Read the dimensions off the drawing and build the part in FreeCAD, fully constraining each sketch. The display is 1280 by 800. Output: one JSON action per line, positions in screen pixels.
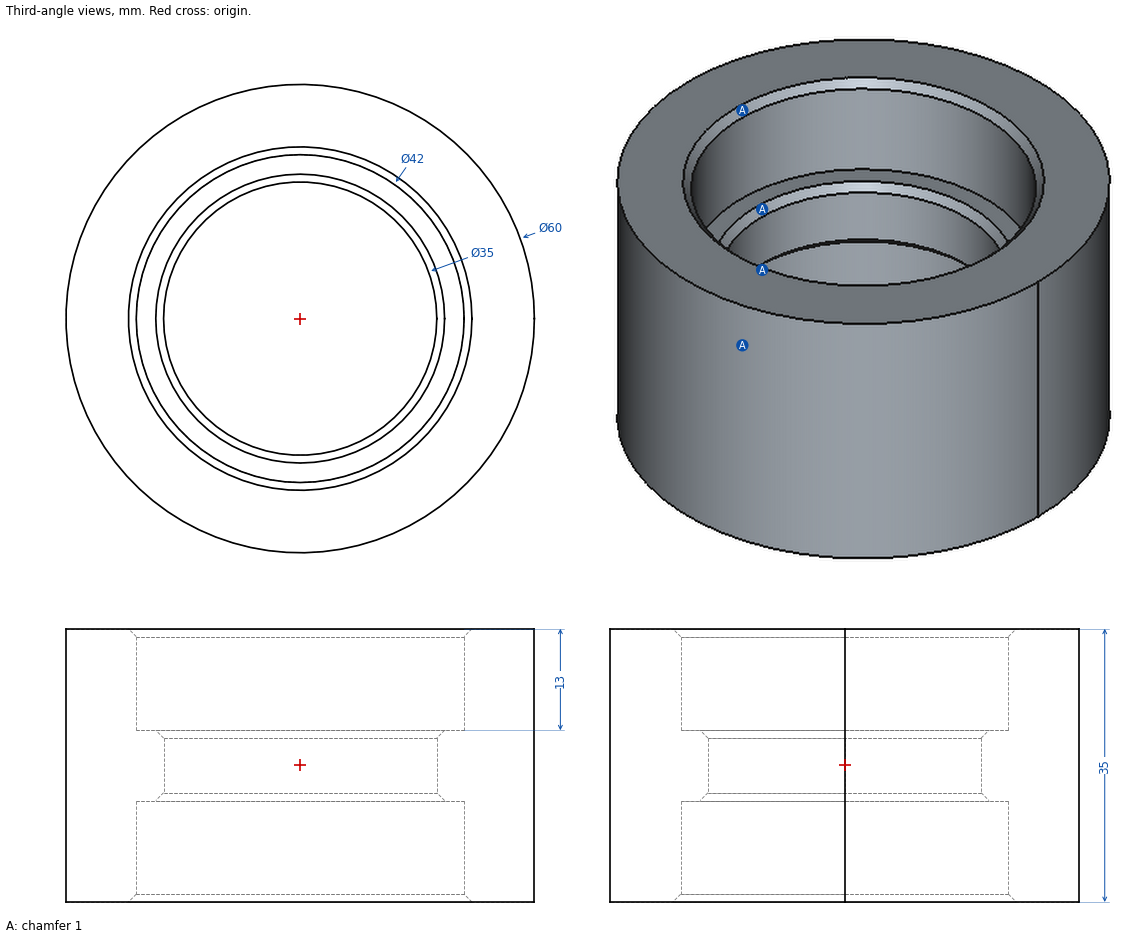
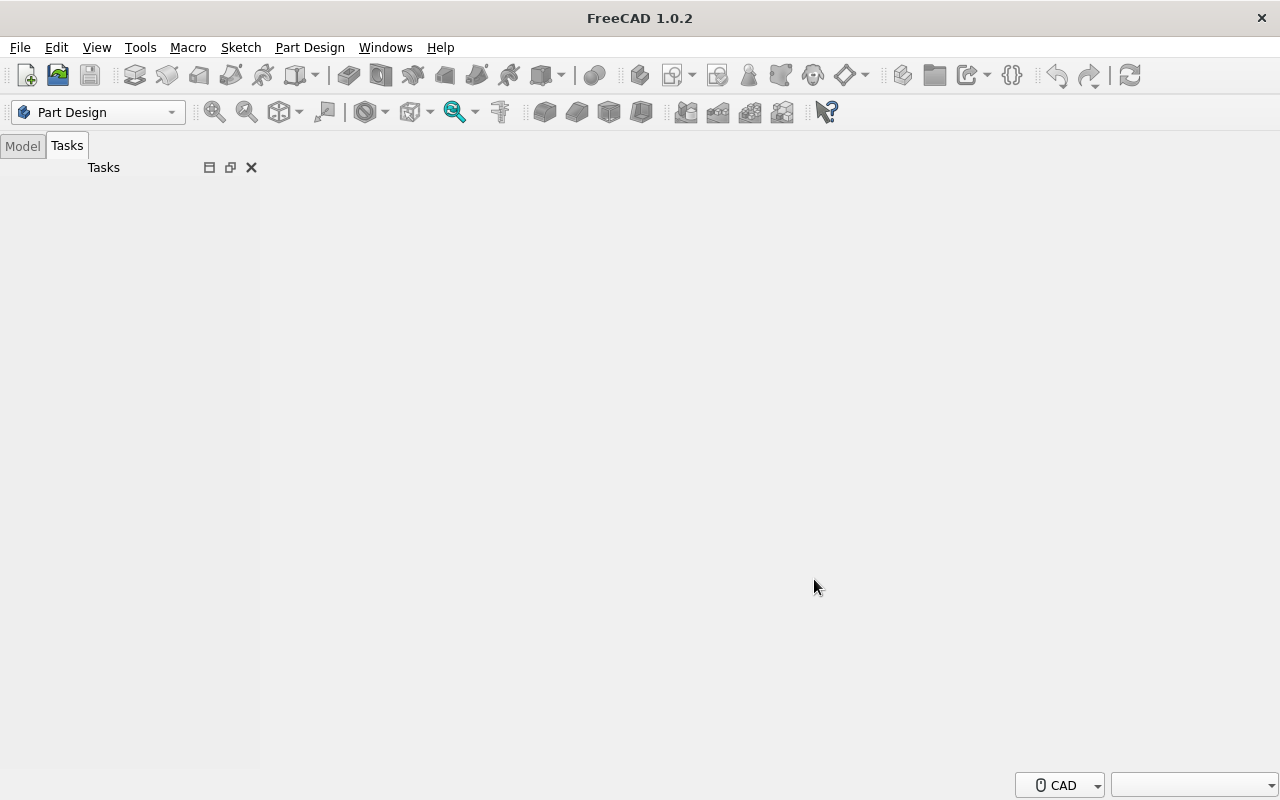
{"action": "left_click", "coordinate": [26, 76]}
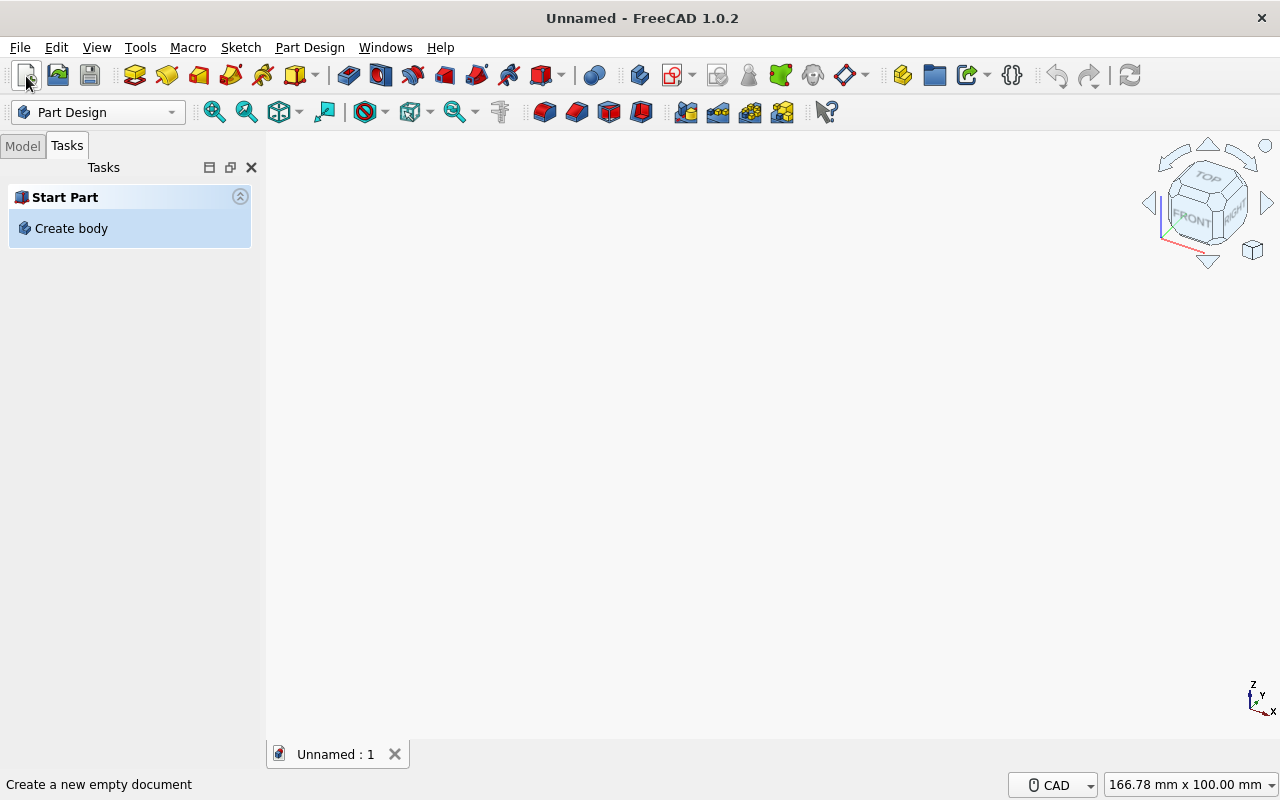
{"action": "left_click", "coordinate": [672, 76]}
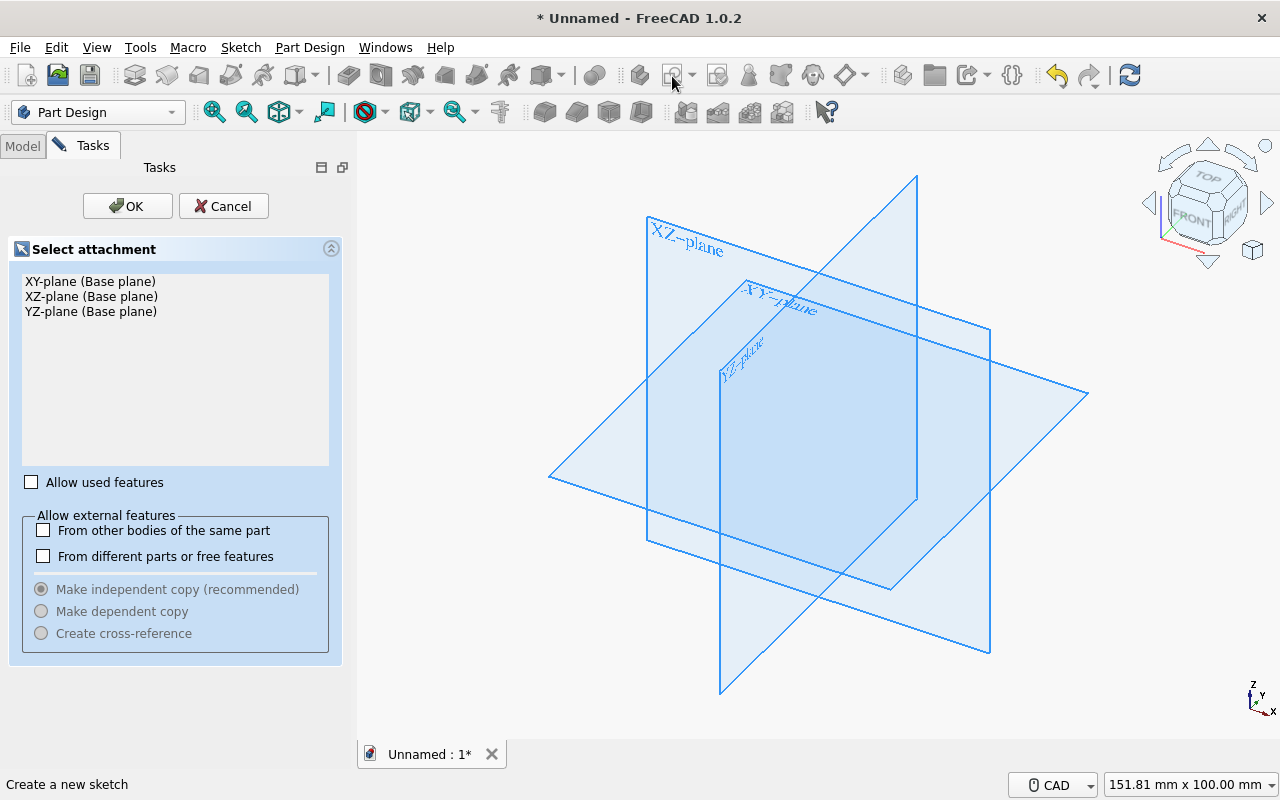
{"action": "left_click", "coordinate": [82, 282]}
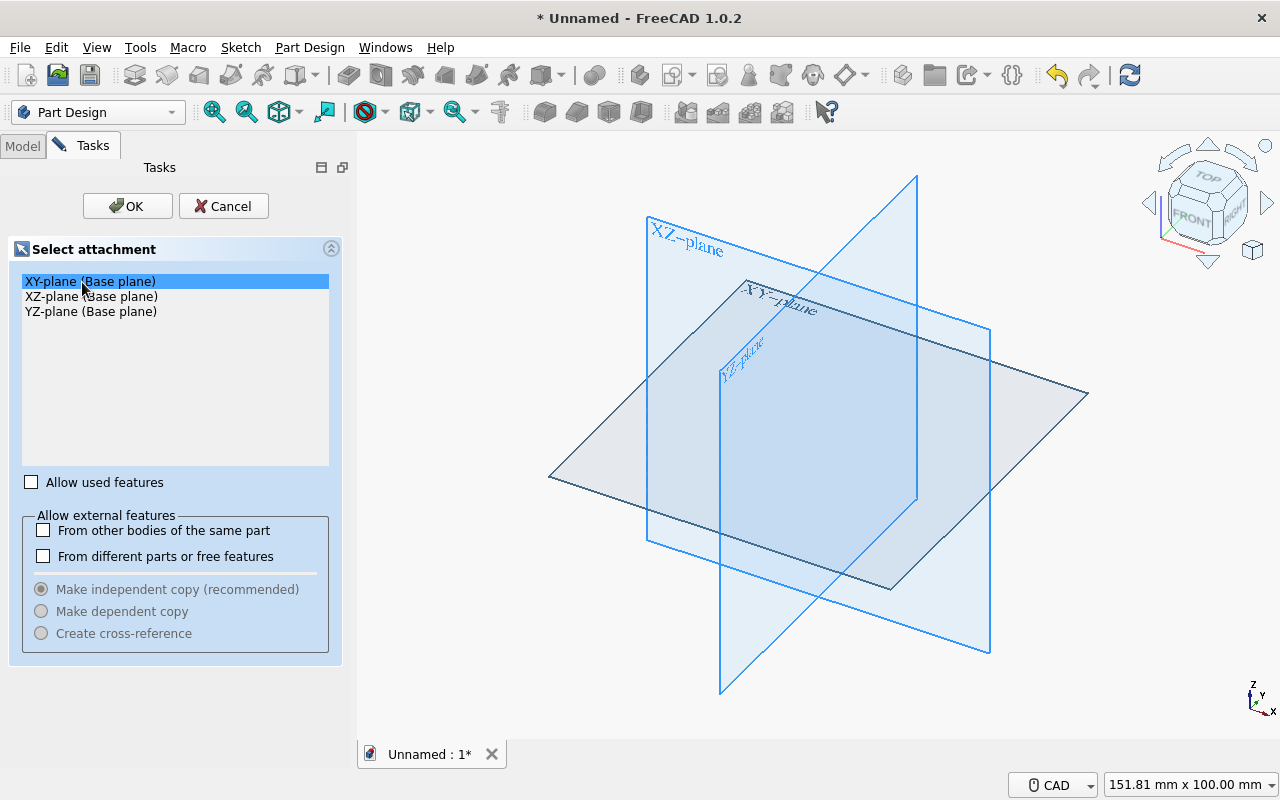
{"action": "left_click", "coordinate": [128, 206]}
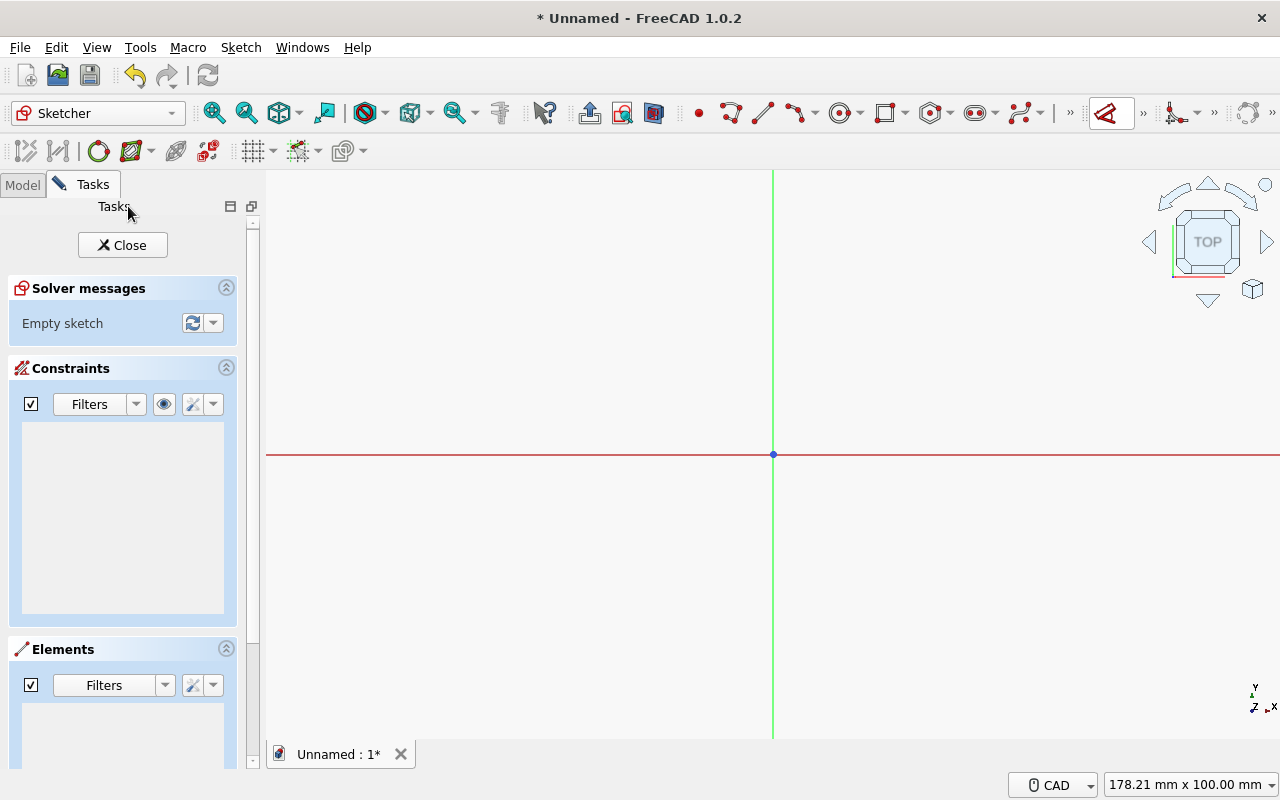
{"action": "key", "text": "g c"}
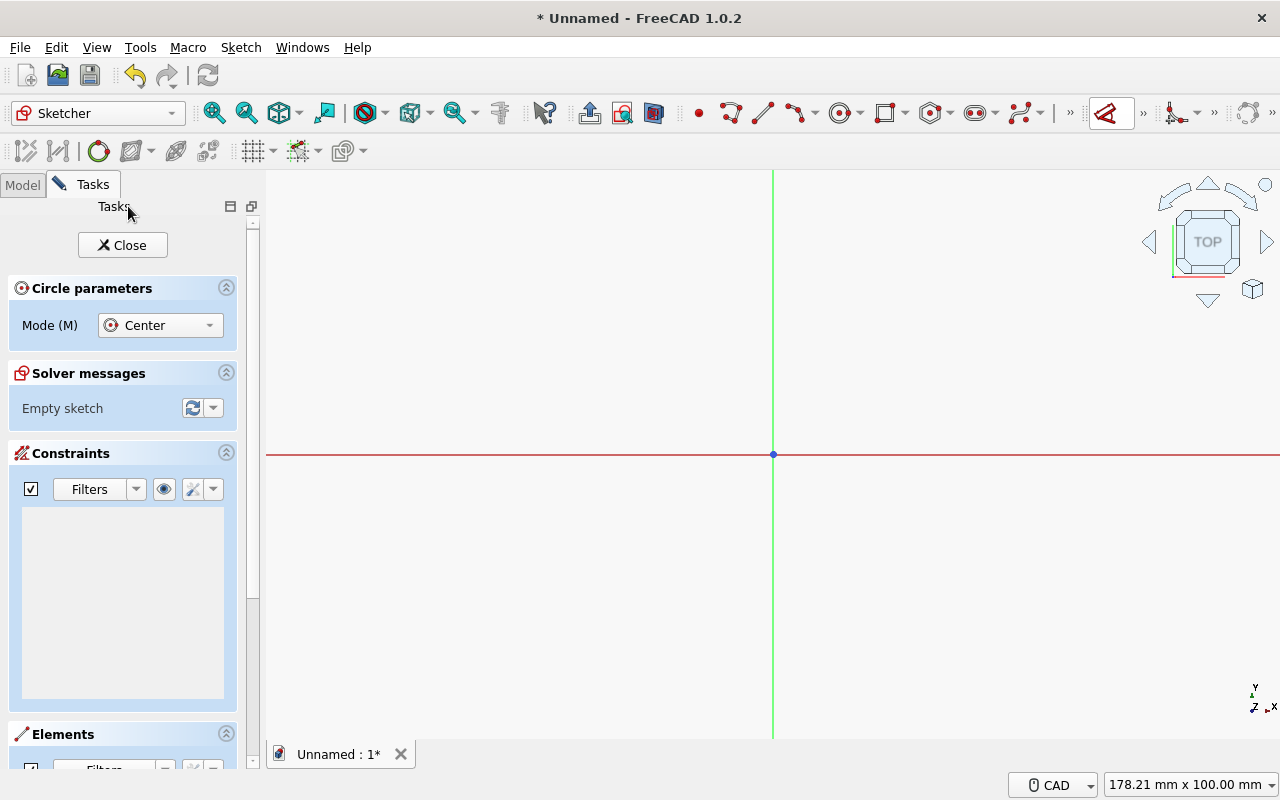
{"action": "left_click", "coordinate": [773, 454]}
{"action": "mouse_move", "coordinate": [894, 334]}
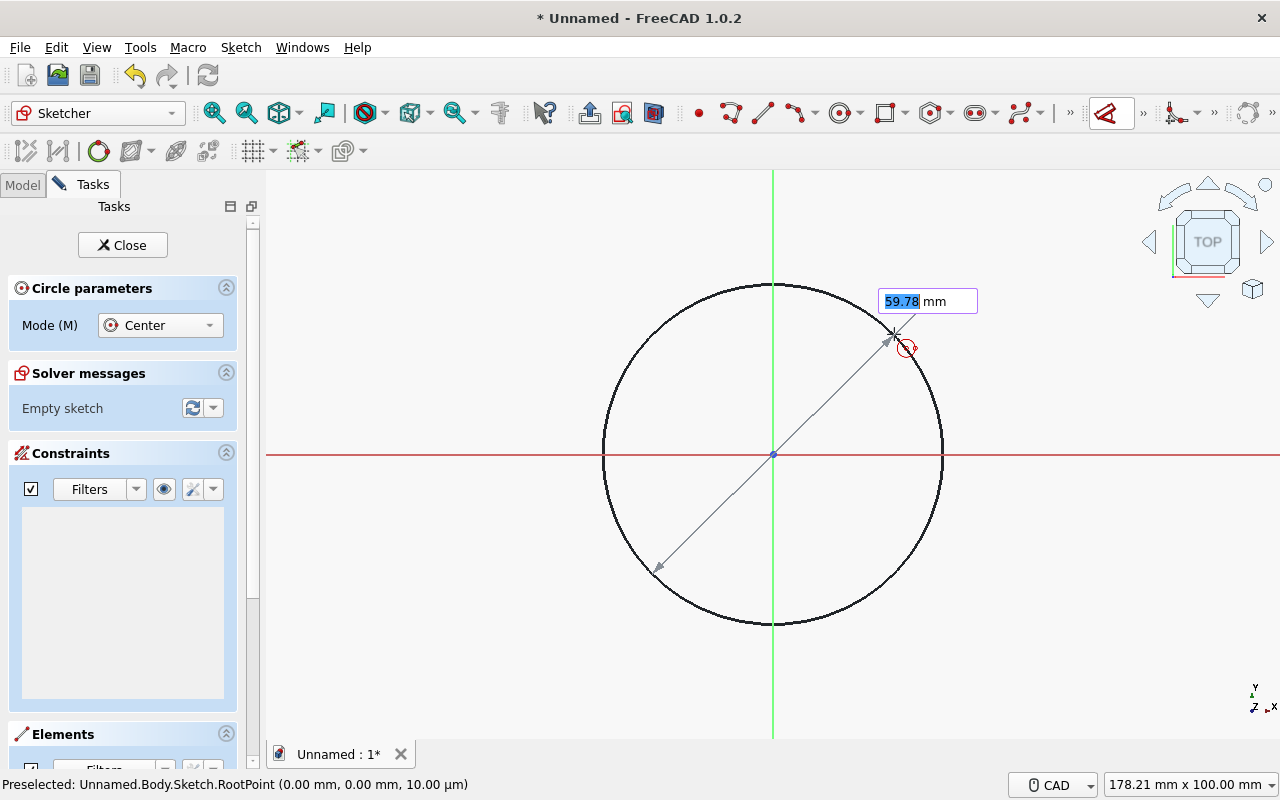
{"action": "type", "text": "60"}
{"action": "key", "text": "Return"}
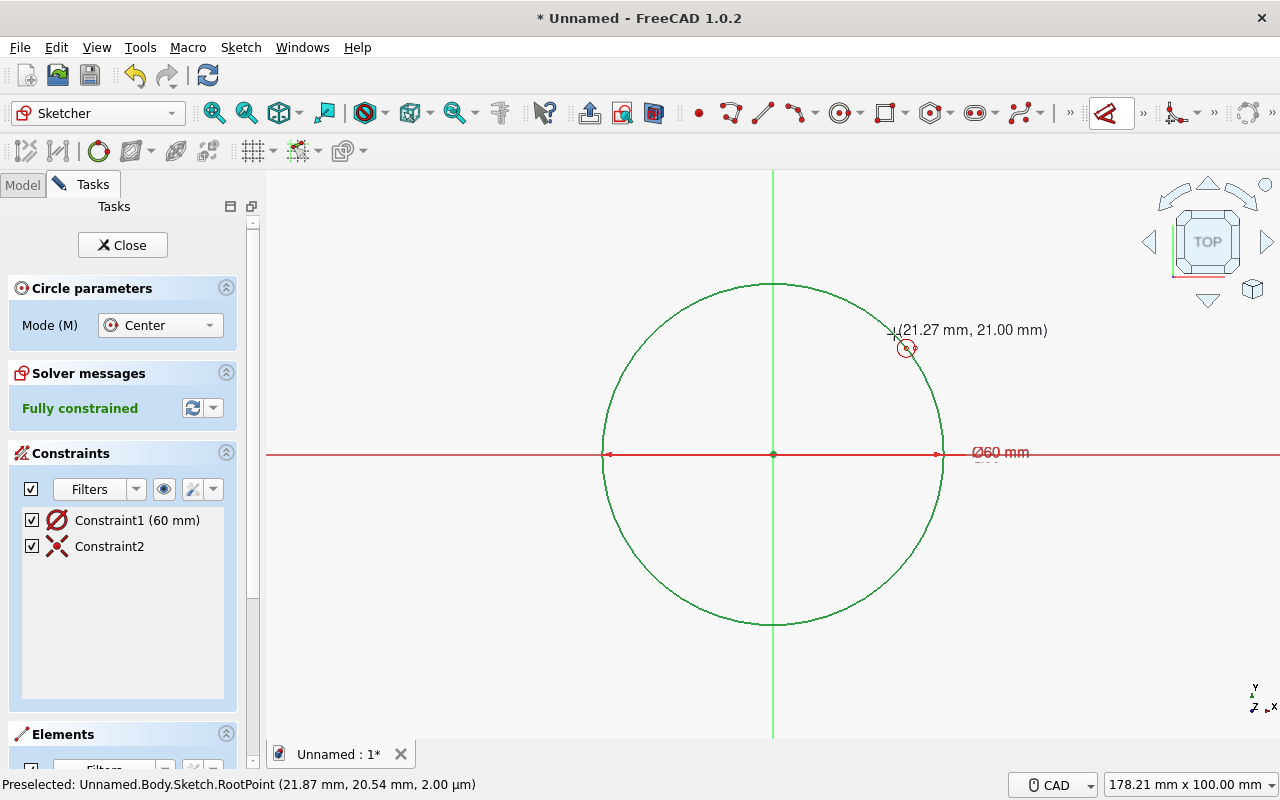
{"action": "left_click", "coordinate": [773, 454]}
{"action": "mouse_move", "coordinate": [843, 384]}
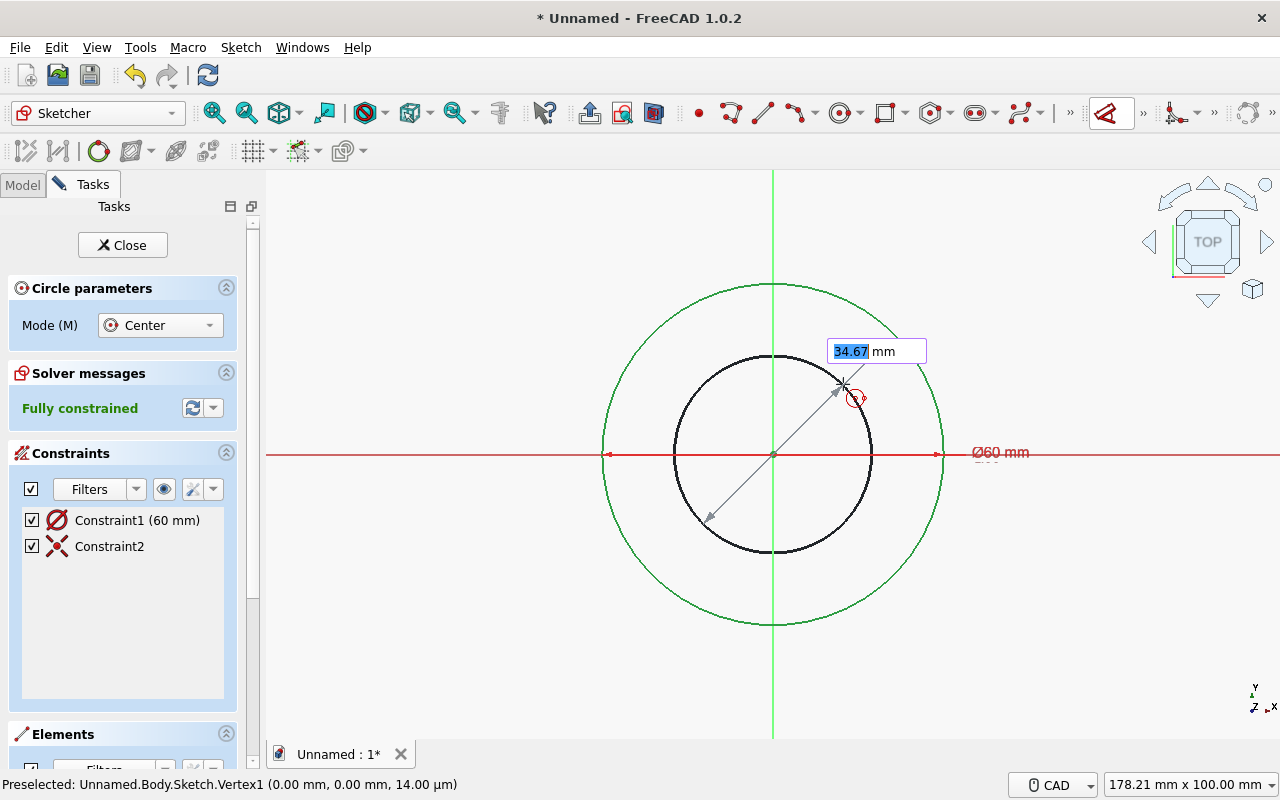
{"action": "type", "text": "35"}
{"action": "key", "text": "Return"}
{"action": "key", "text": "Escape"}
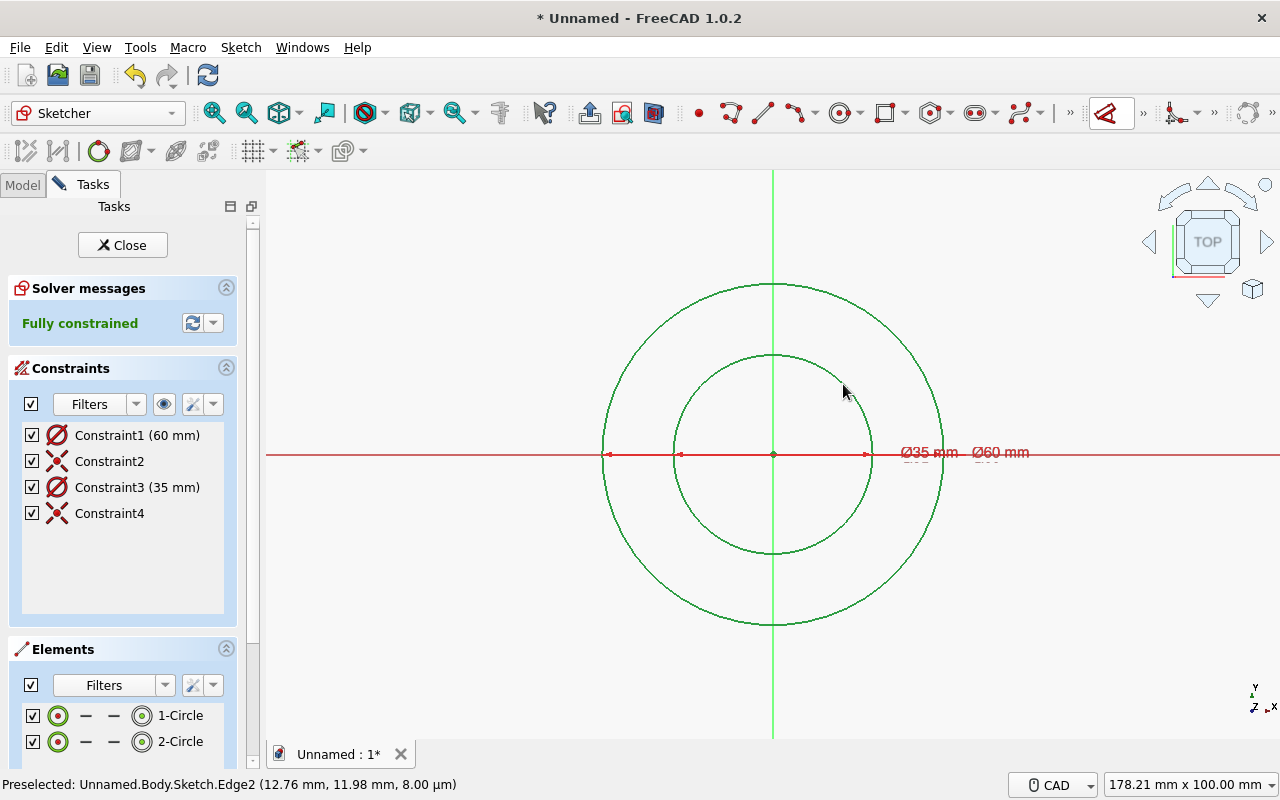
{"action": "left_click", "coordinate": [123, 245]}